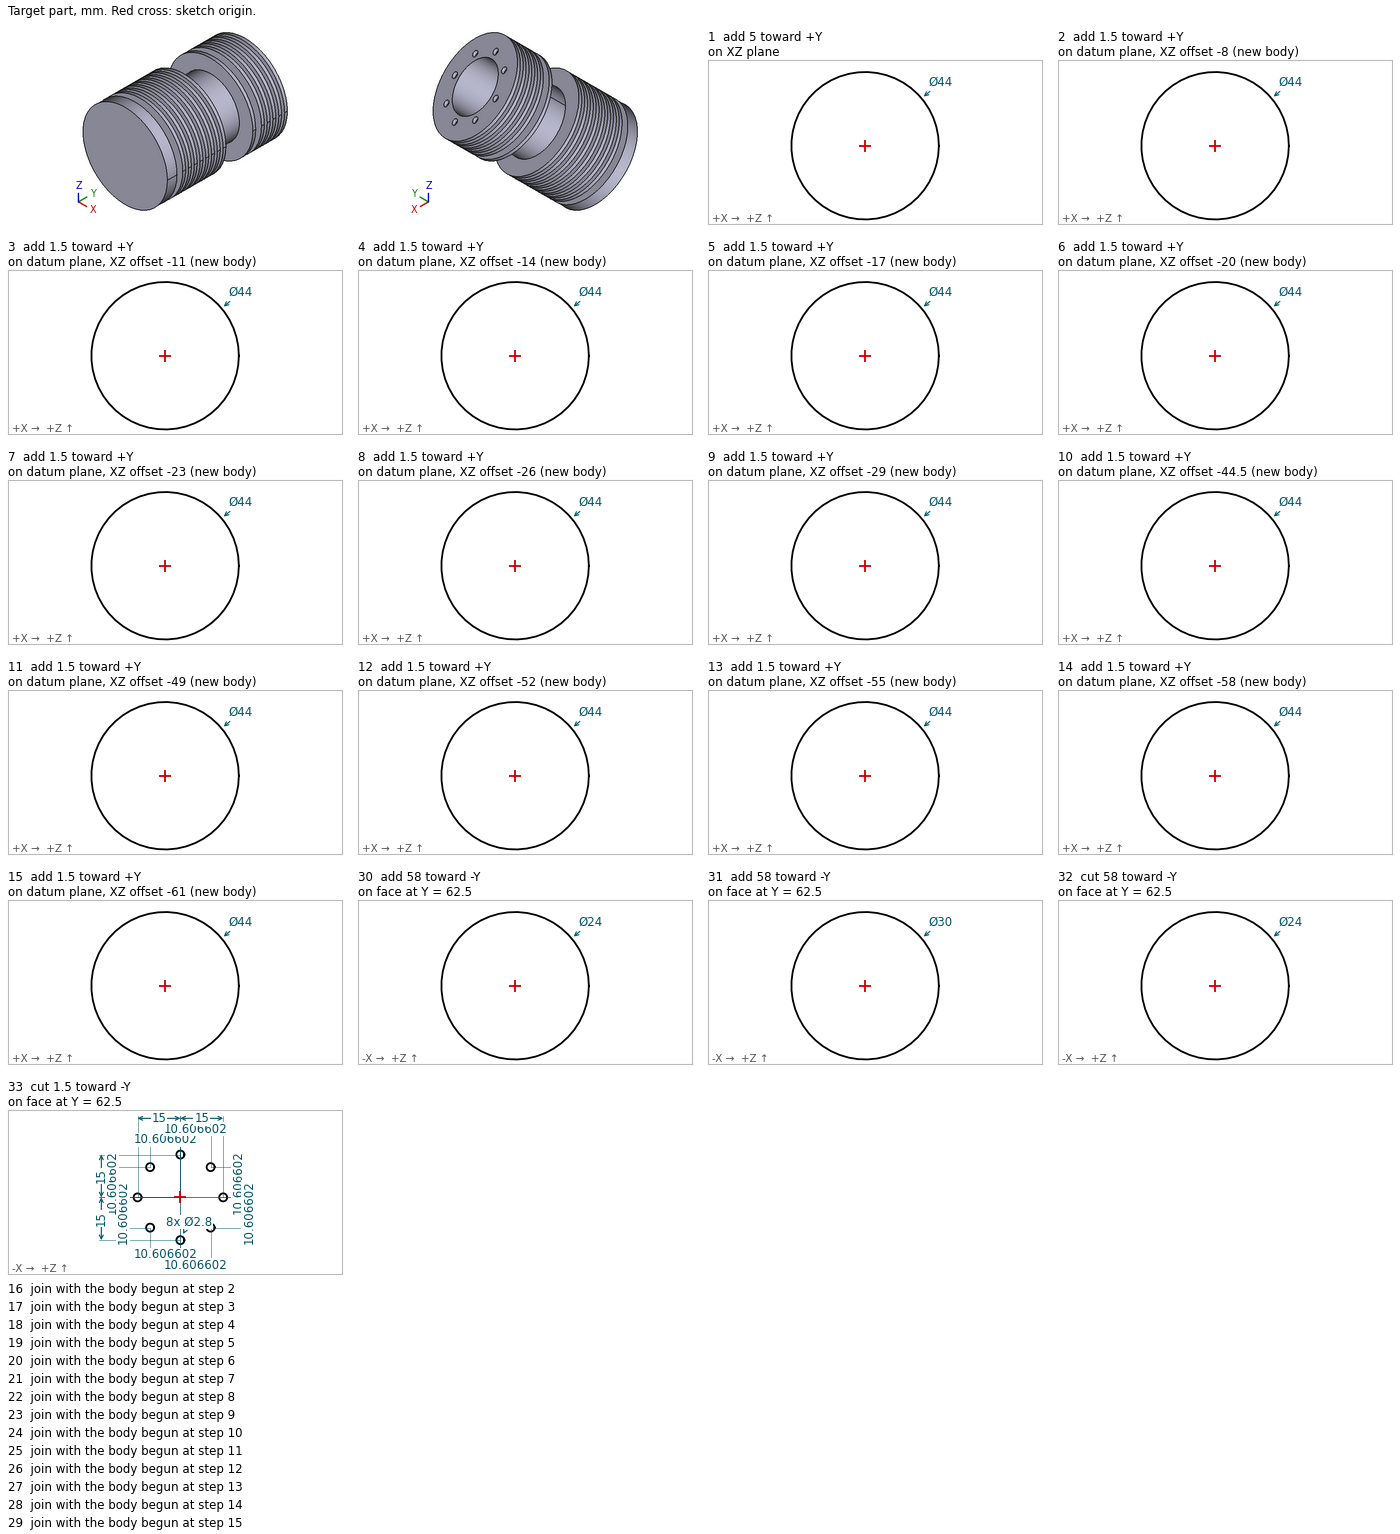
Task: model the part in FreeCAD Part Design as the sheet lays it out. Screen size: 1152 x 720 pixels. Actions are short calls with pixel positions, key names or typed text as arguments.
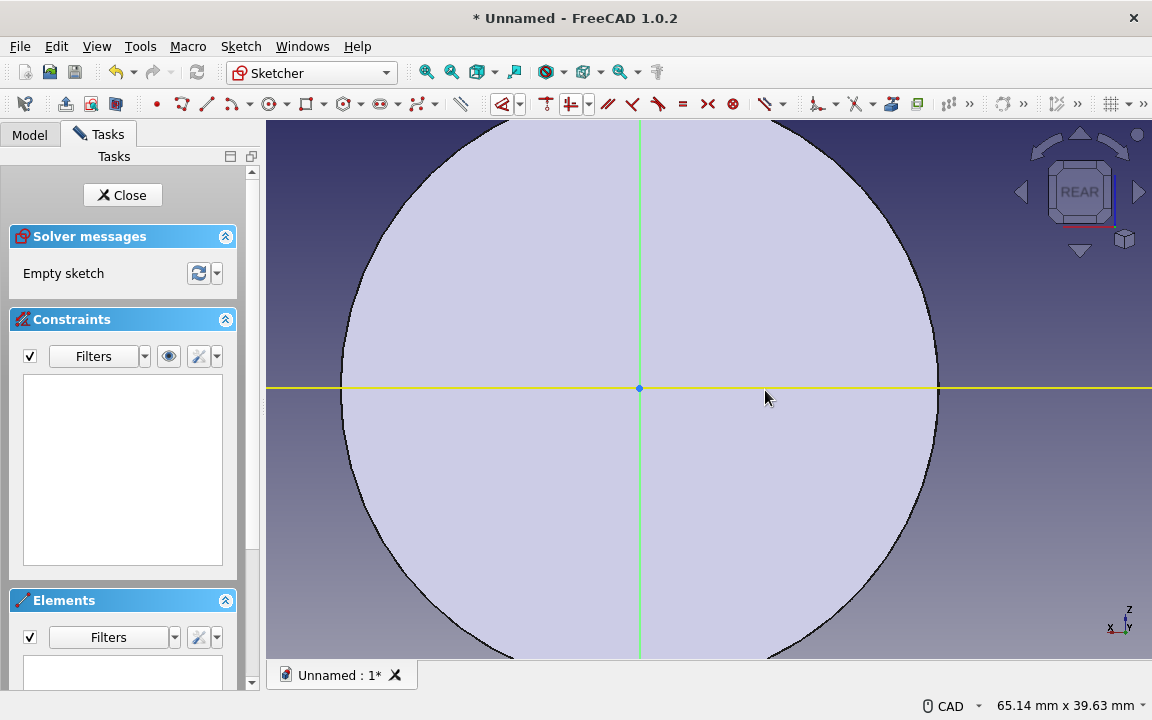
key(g)
key(c)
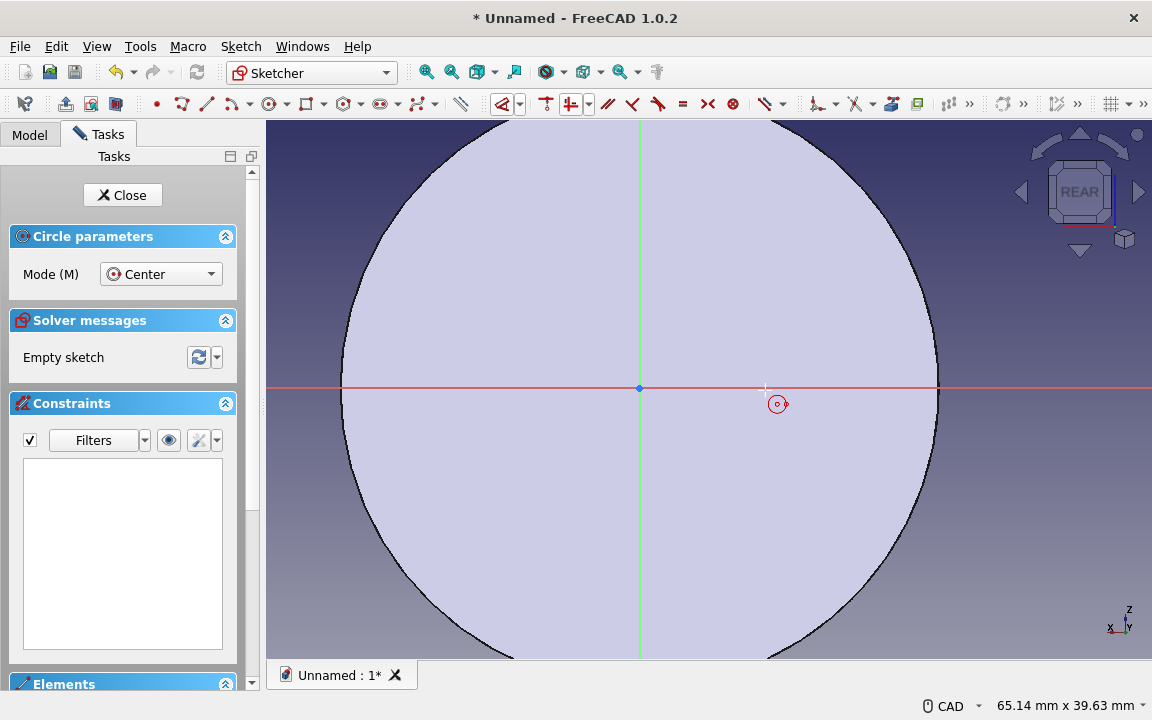
click(640, 388)
click(755, 273)
key(Escape)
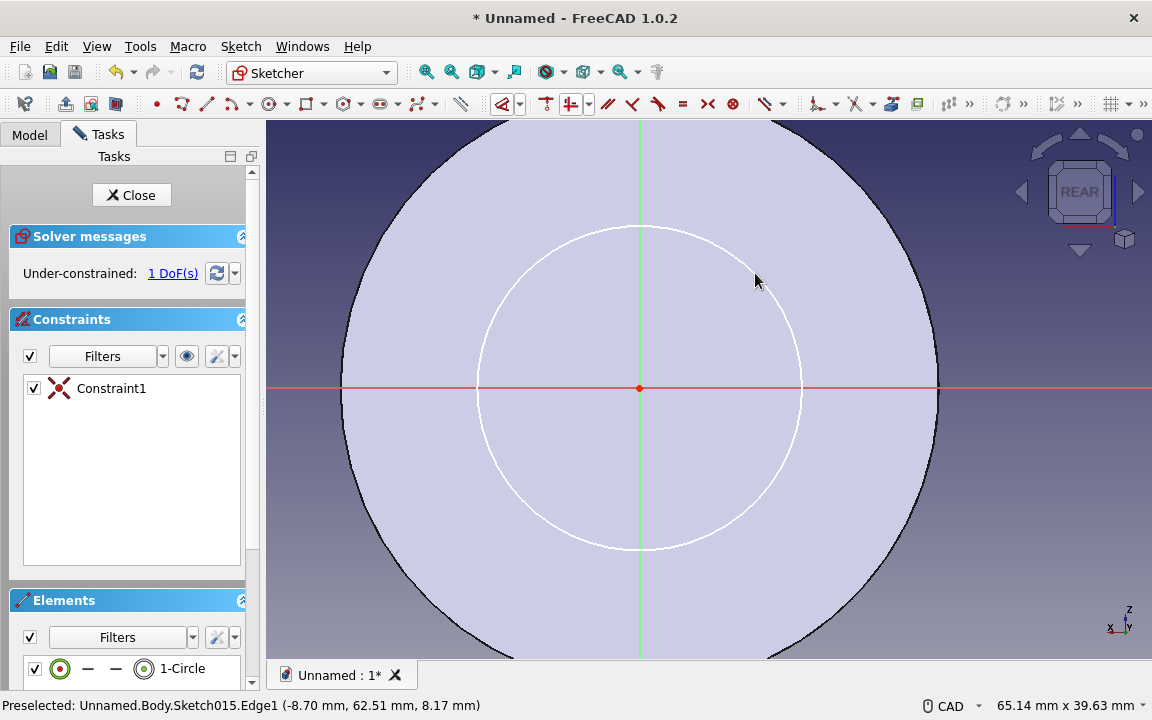
click(754, 273)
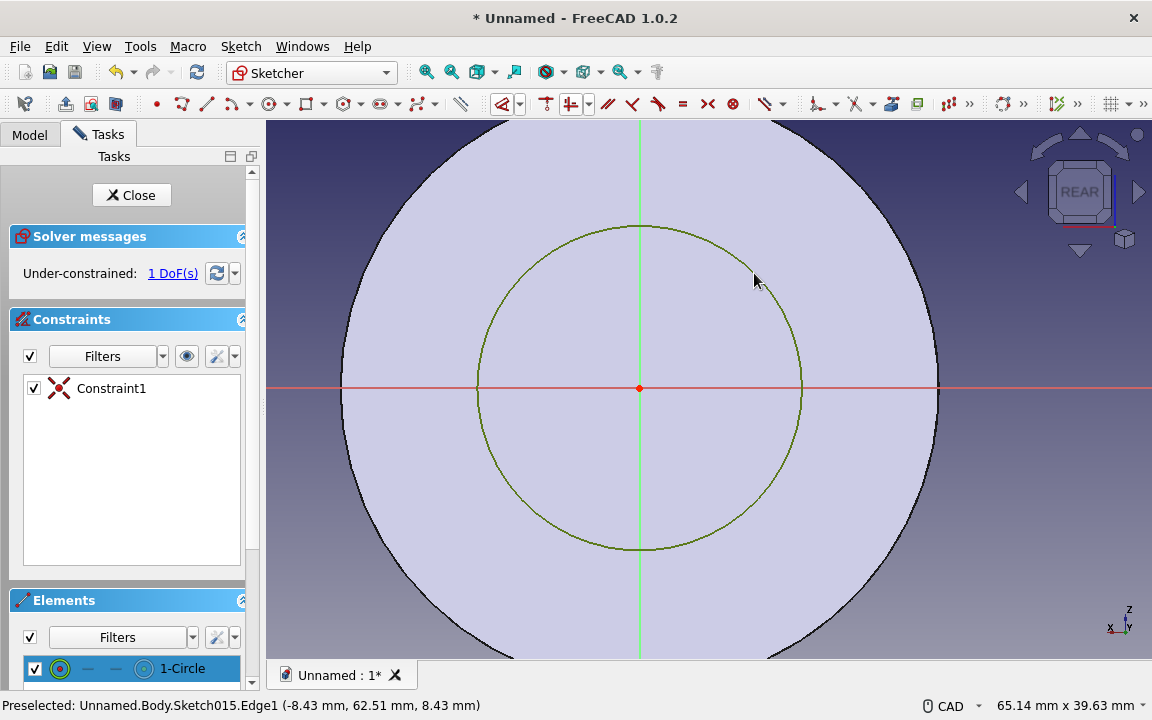
click(520, 104)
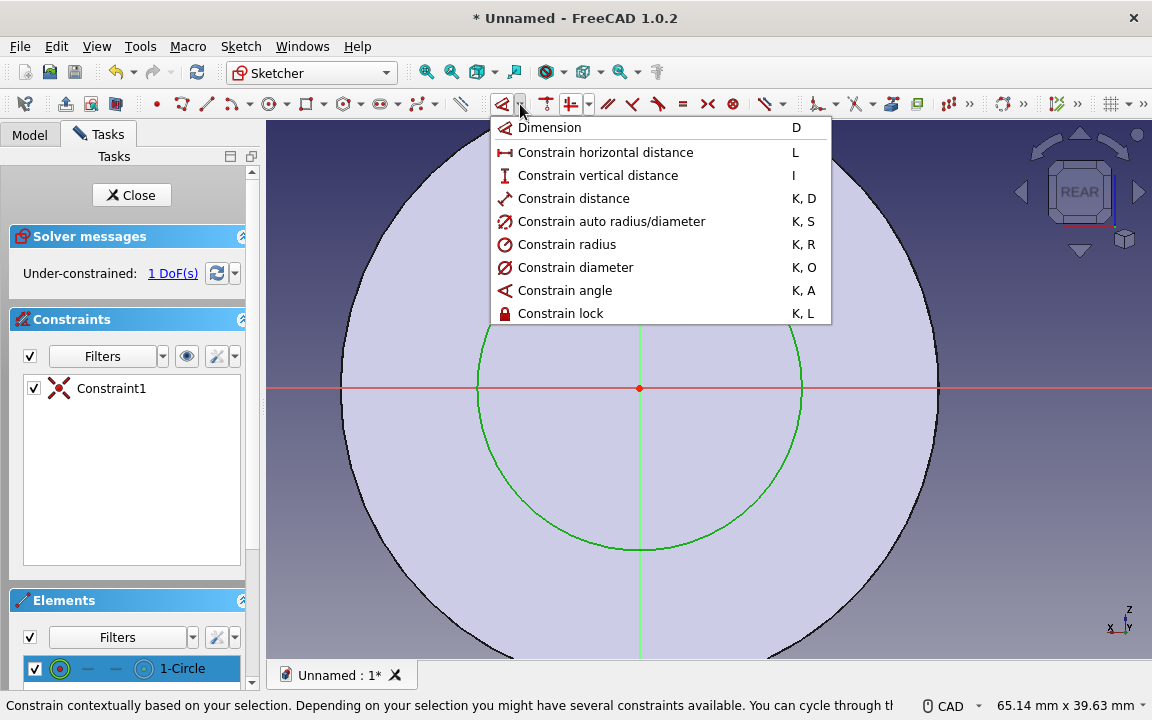
click(661, 268)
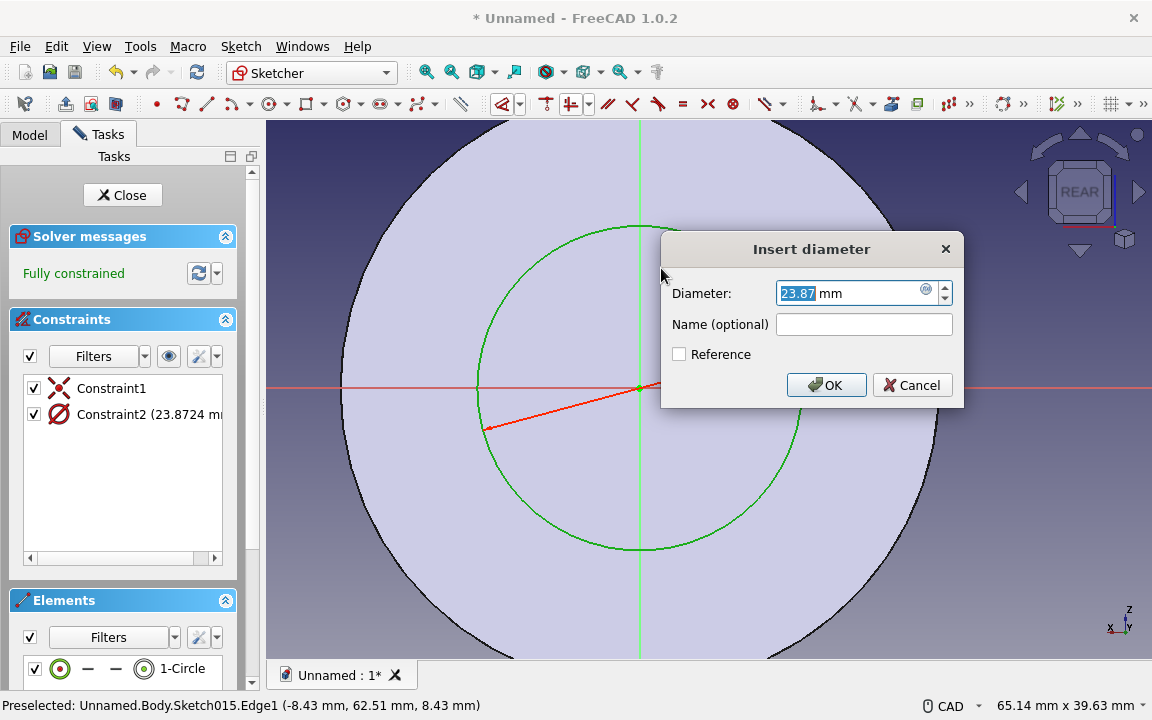
text(24)
key(Return)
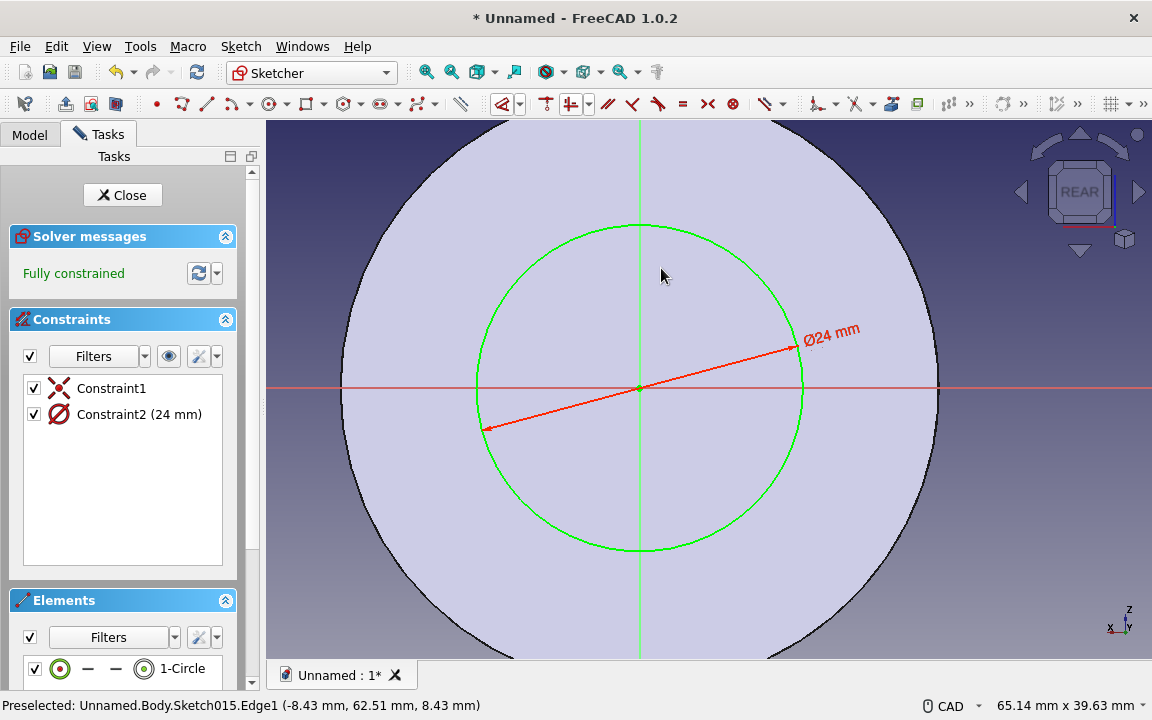
click(123, 195)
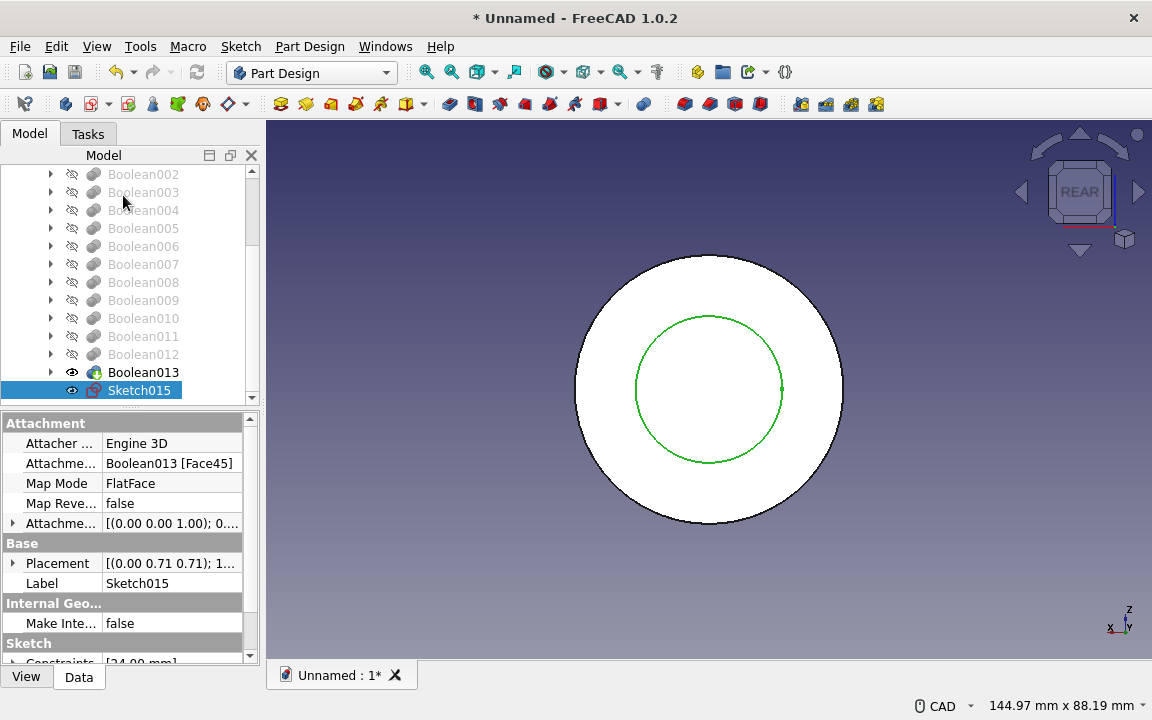
click(281, 104)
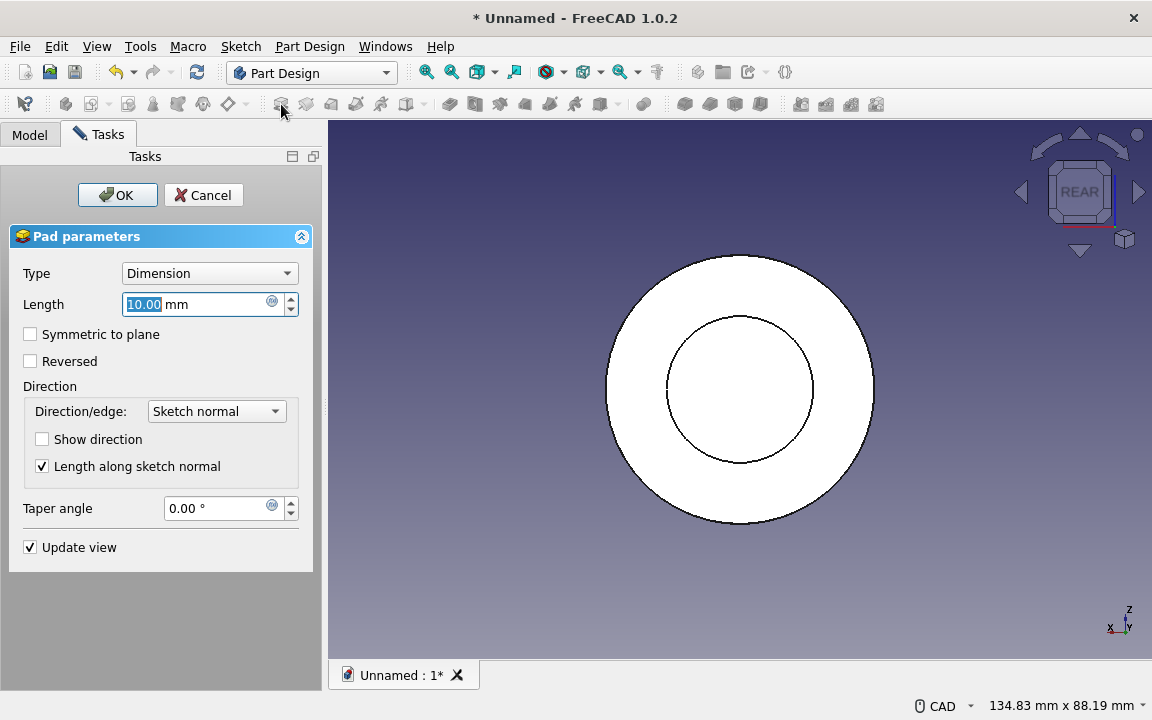
text(58)
key(Tab)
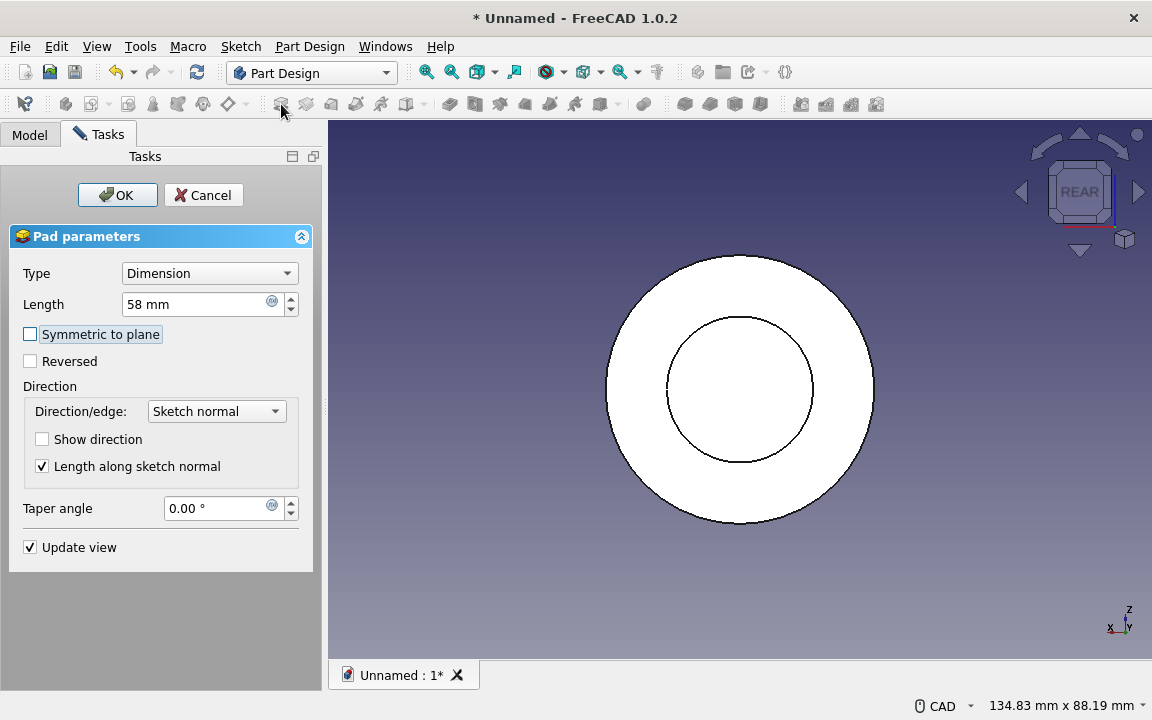
click(31, 361)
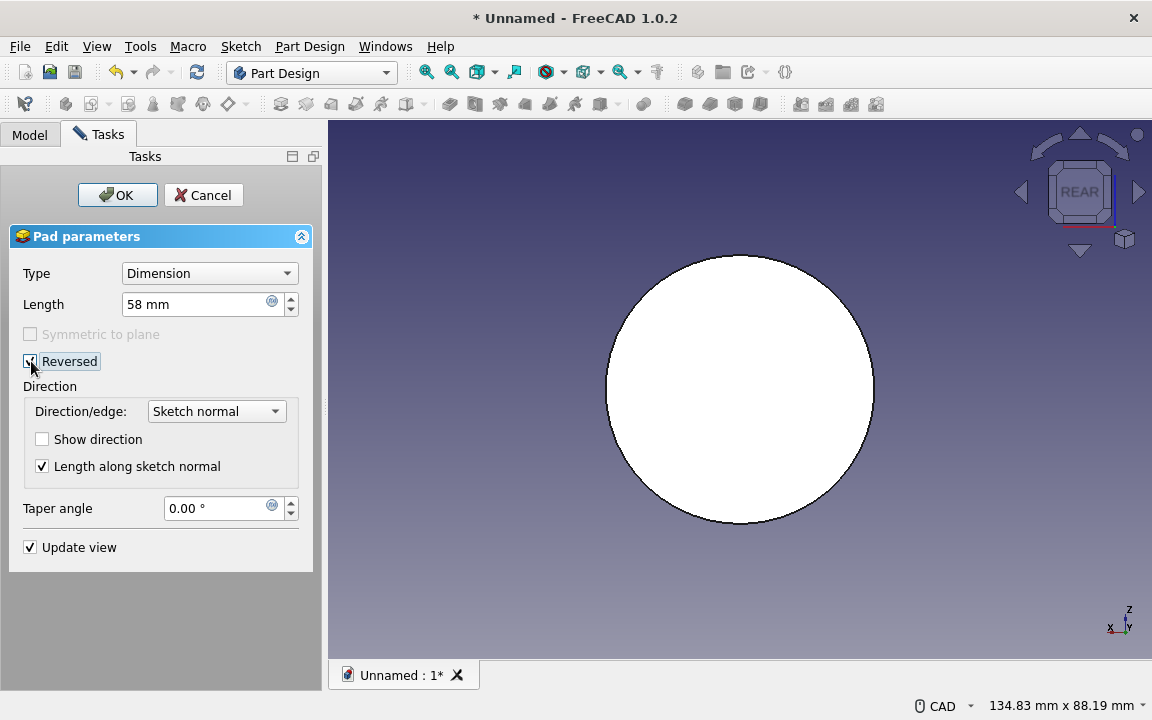
click(118, 195)